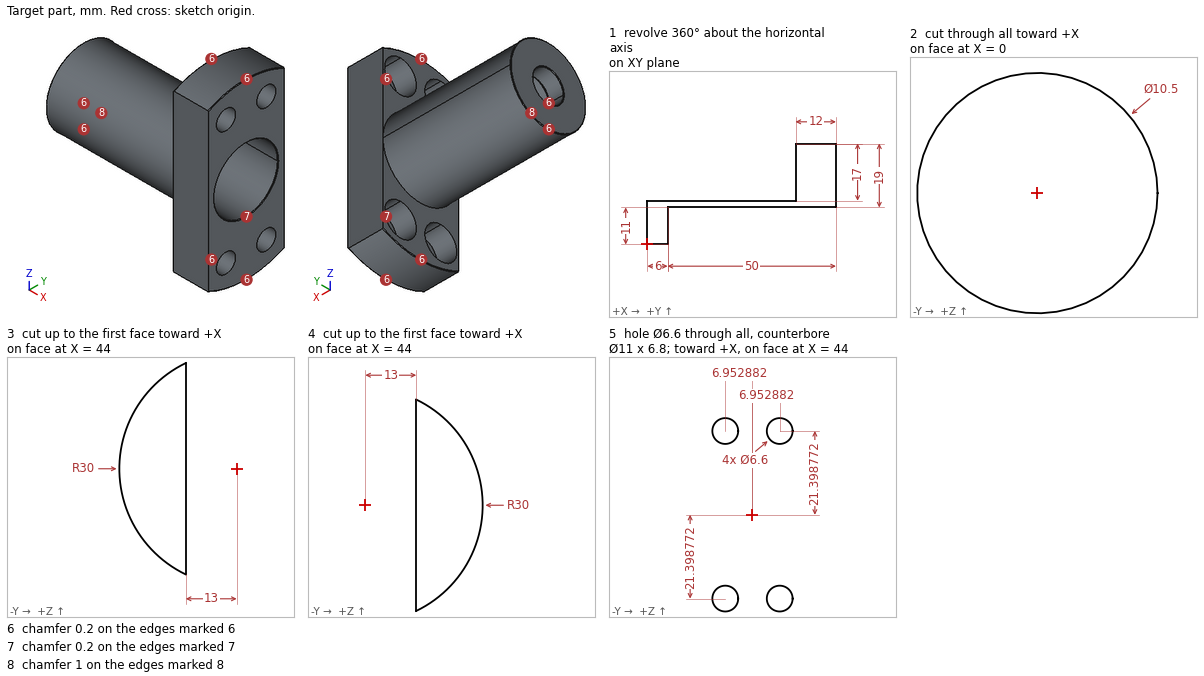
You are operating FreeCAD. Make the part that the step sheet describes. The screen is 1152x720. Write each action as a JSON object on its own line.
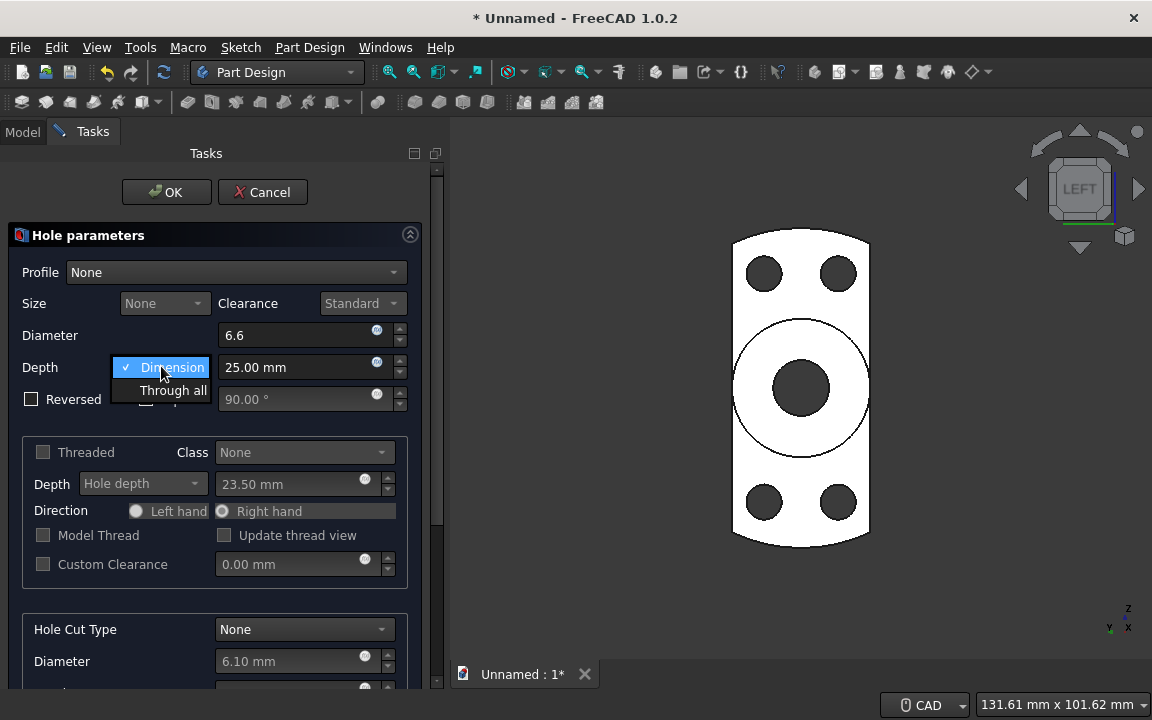
{"action": "left_click", "coordinate": [160, 390]}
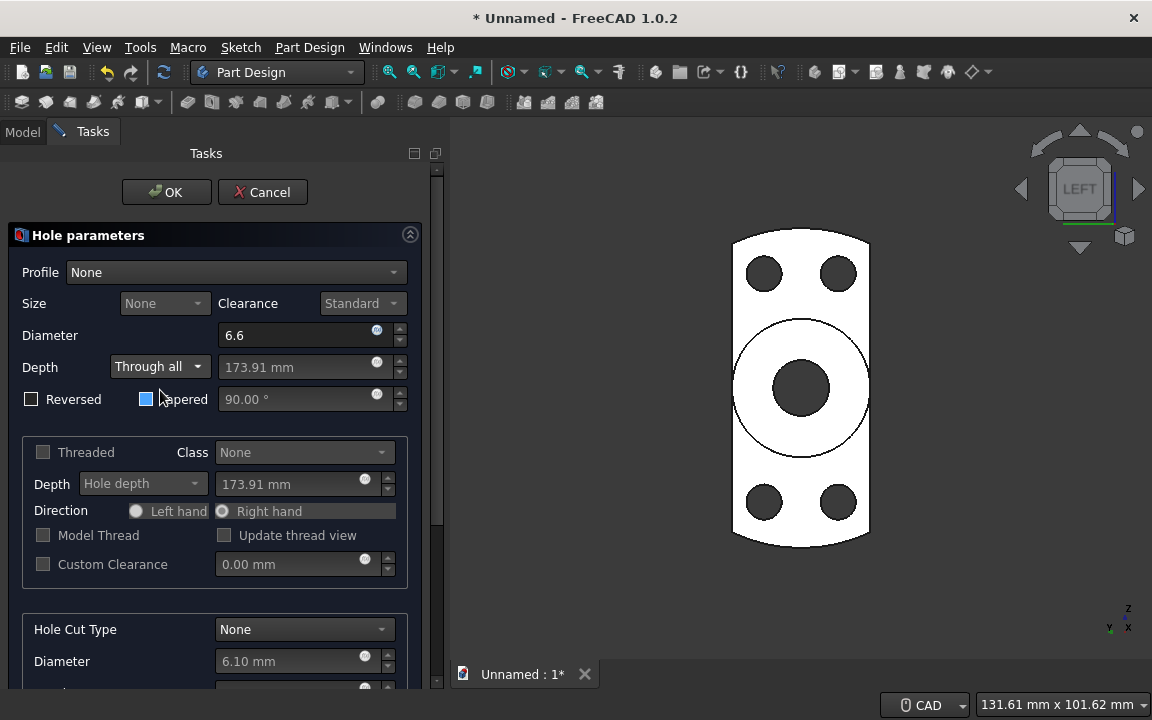
{"action": "left_click", "coordinate": [306, 630]}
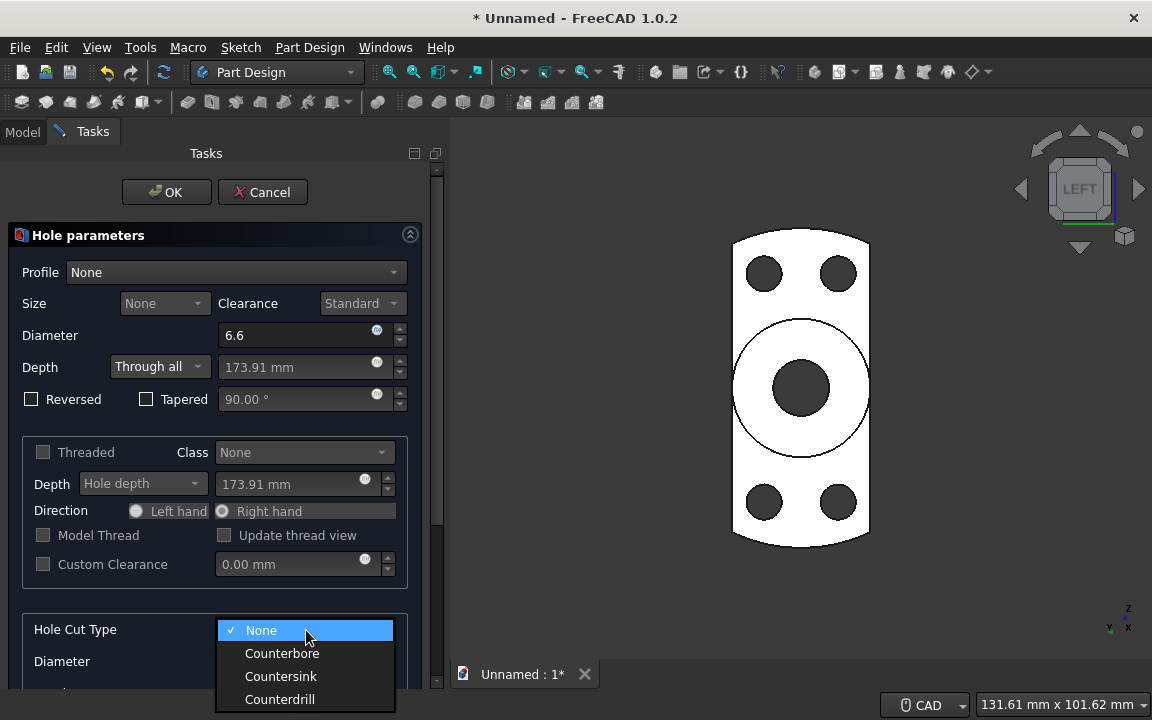
{"action": "left_click", "coordinate": [304, 654]}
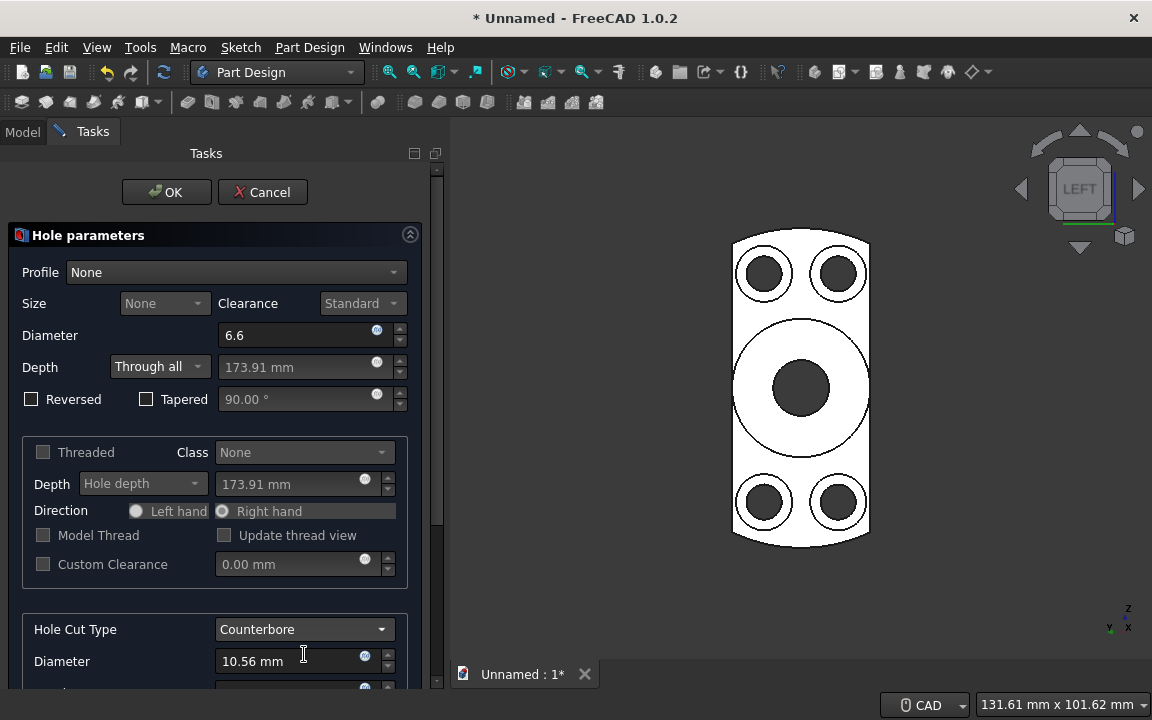
{"action": "triple_click", "coordinate": [298, 661]}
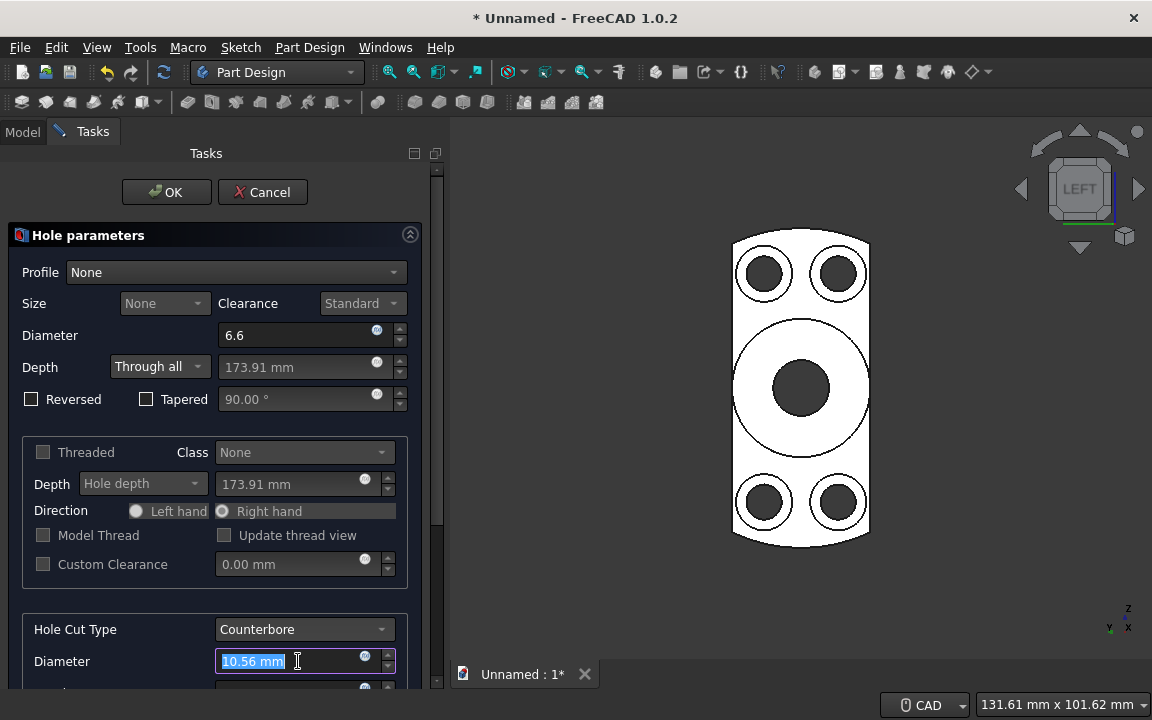
{"action": "type", "text": "11"}
{"action": "key", "text": "Tab"}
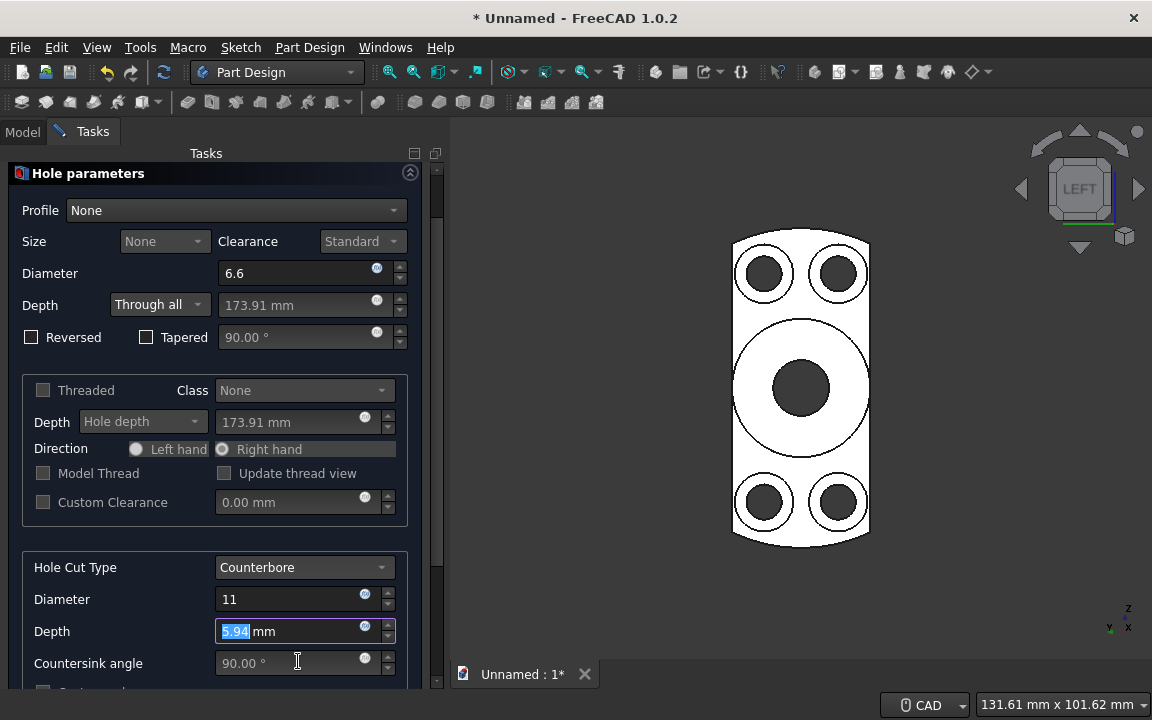
{"action": "type", "text": "6.8"}
{"action": "key", "text": "Tab"}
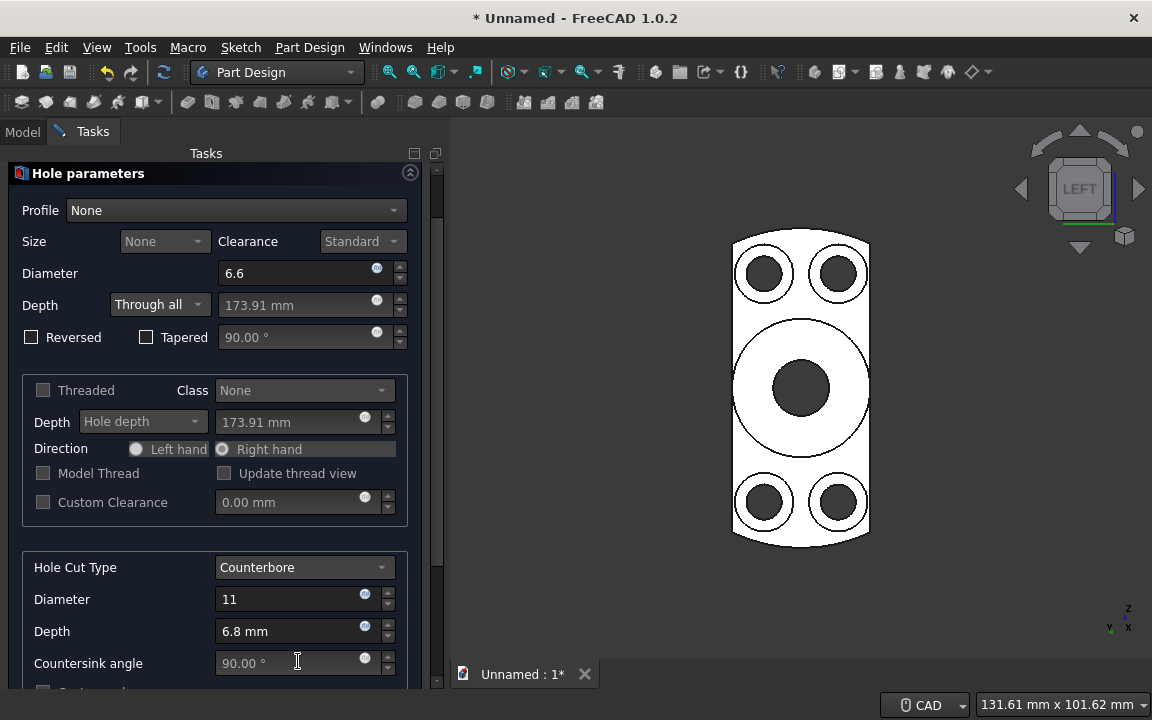
{"action": "scroll", "coordinate": [437, 426], "scroll_direction": "up", "scroll_amount": 2}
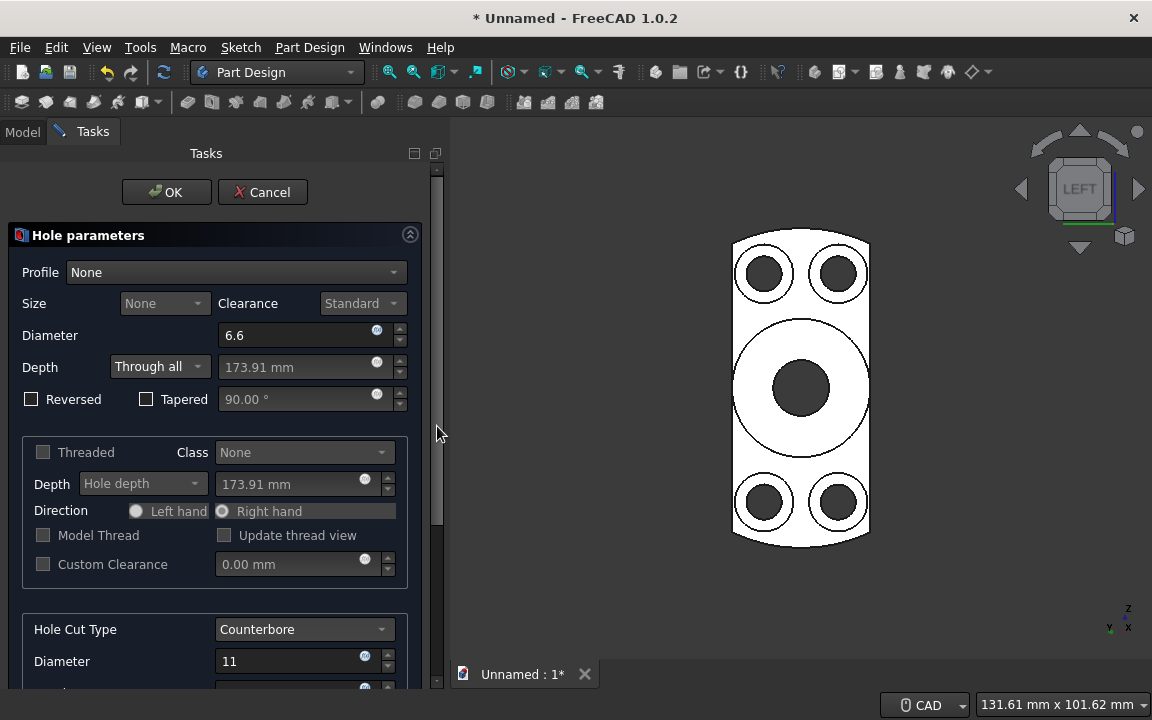
{"action": "left_click", "coordinate": [167, 192]}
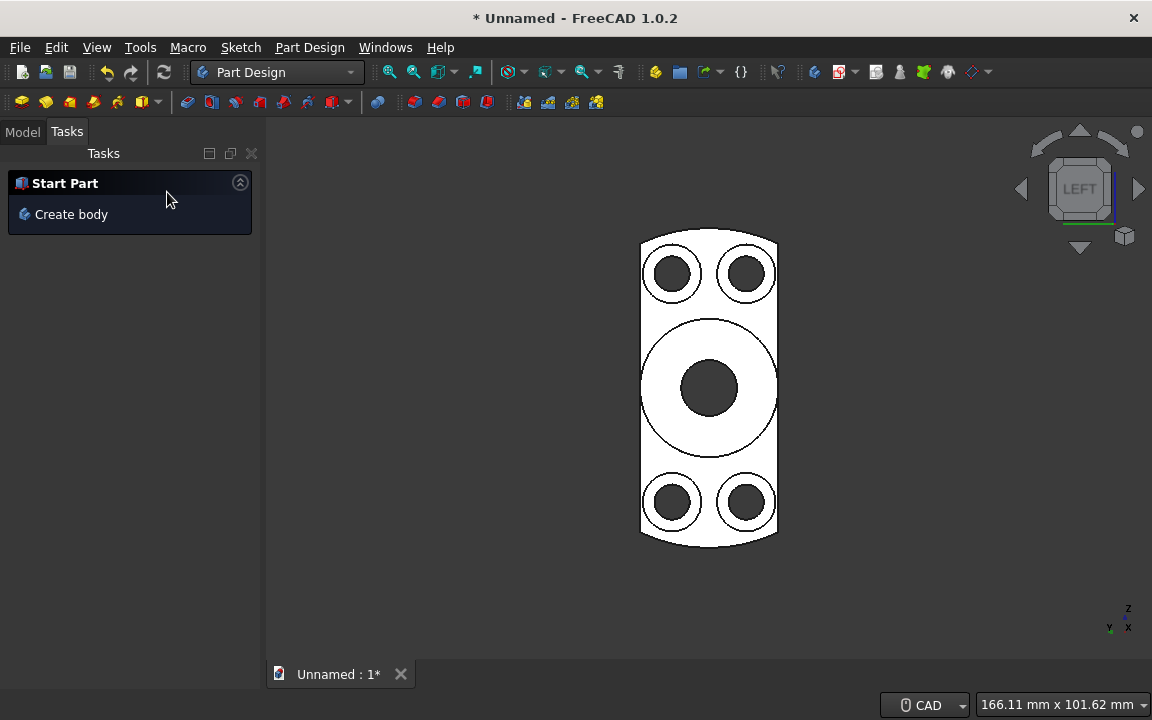
{"action": "left_click", "coordinate": [681, 387]}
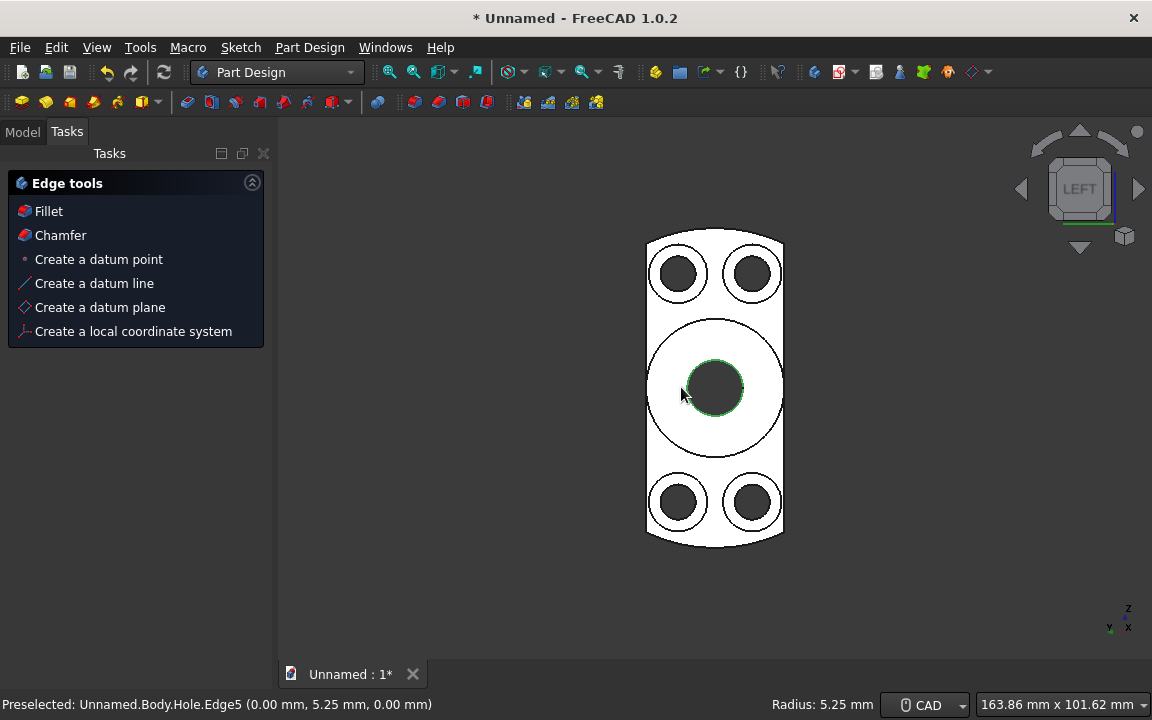
{"action": "left_click", "coordinate": [715, 227], "text": "ctrl"}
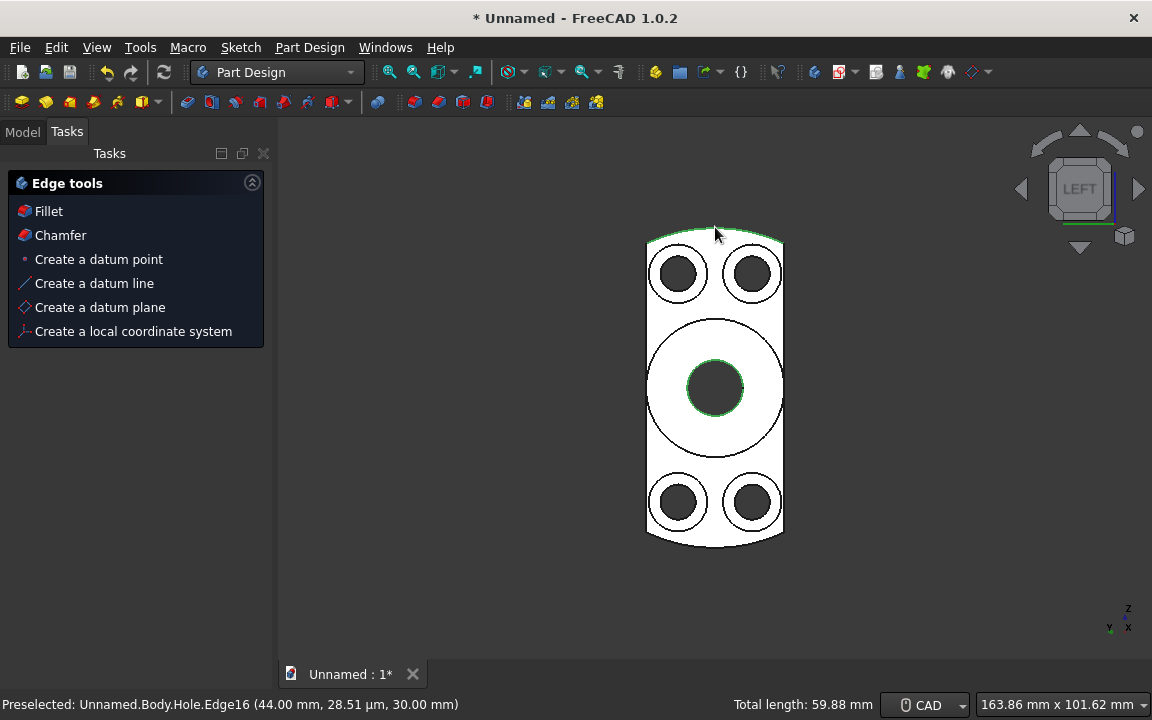
{"action": "left_click", "coordinate": [715, 547], "text": "ctrl"}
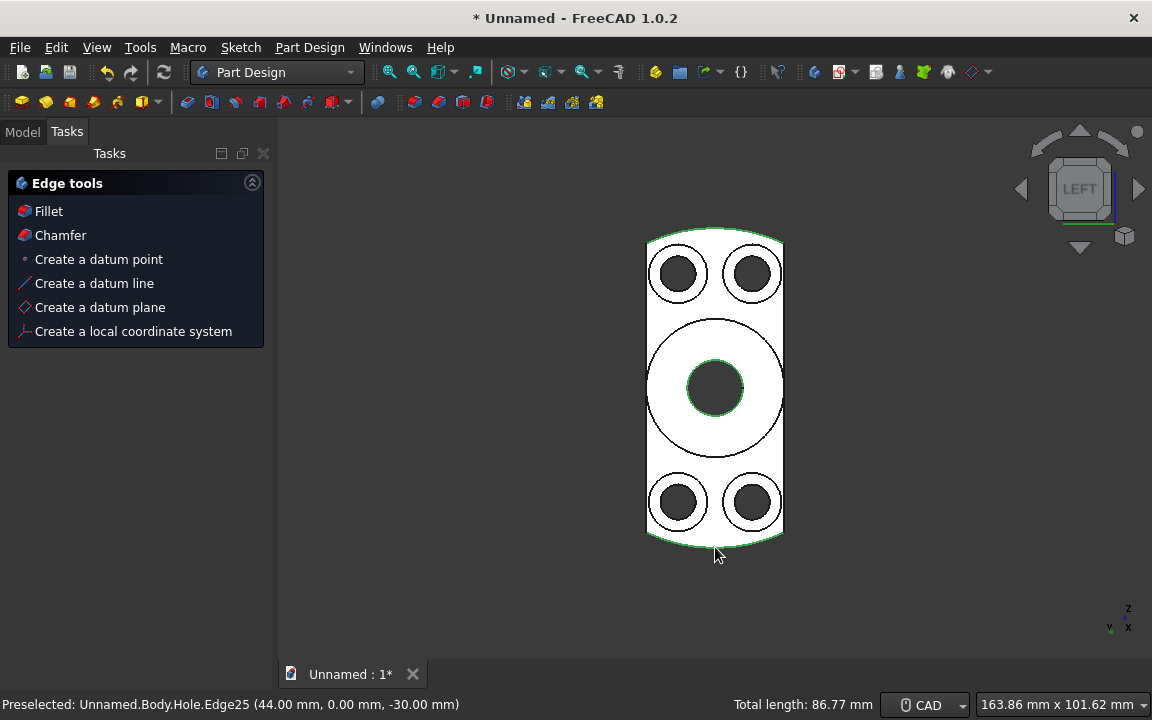
{"action": "left_click", "coordinate": [784, 387], "text": "ctrl"}